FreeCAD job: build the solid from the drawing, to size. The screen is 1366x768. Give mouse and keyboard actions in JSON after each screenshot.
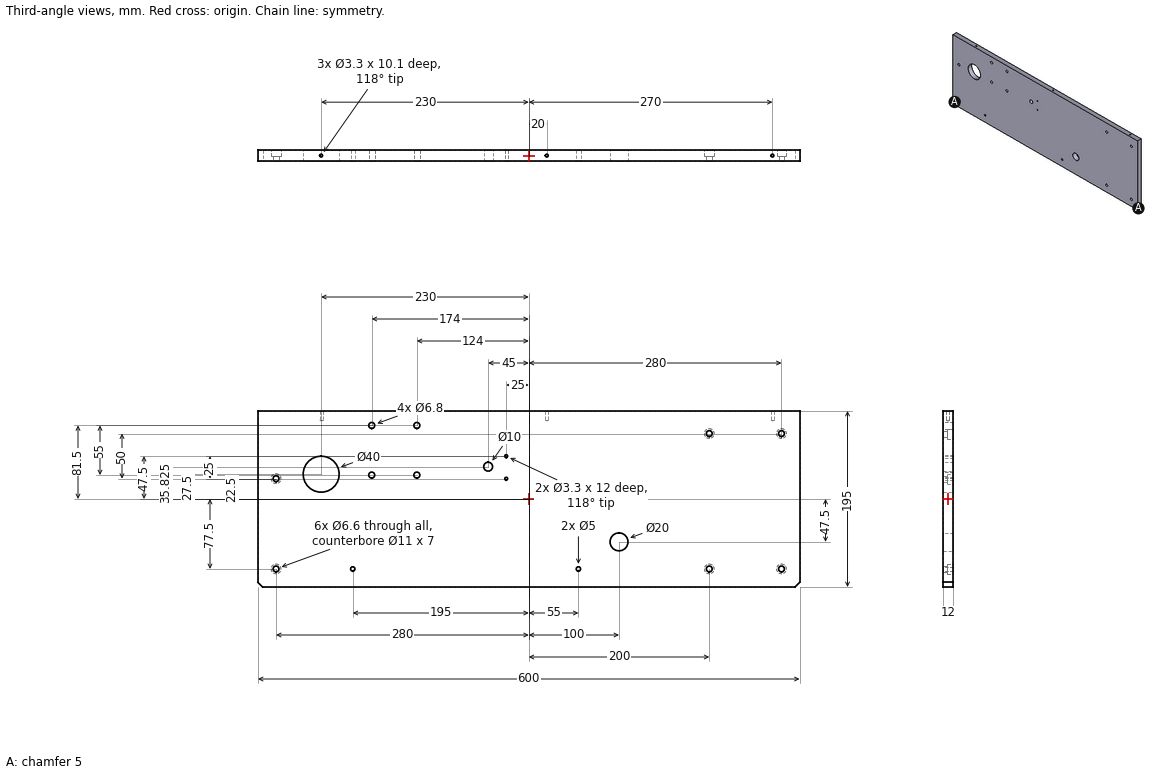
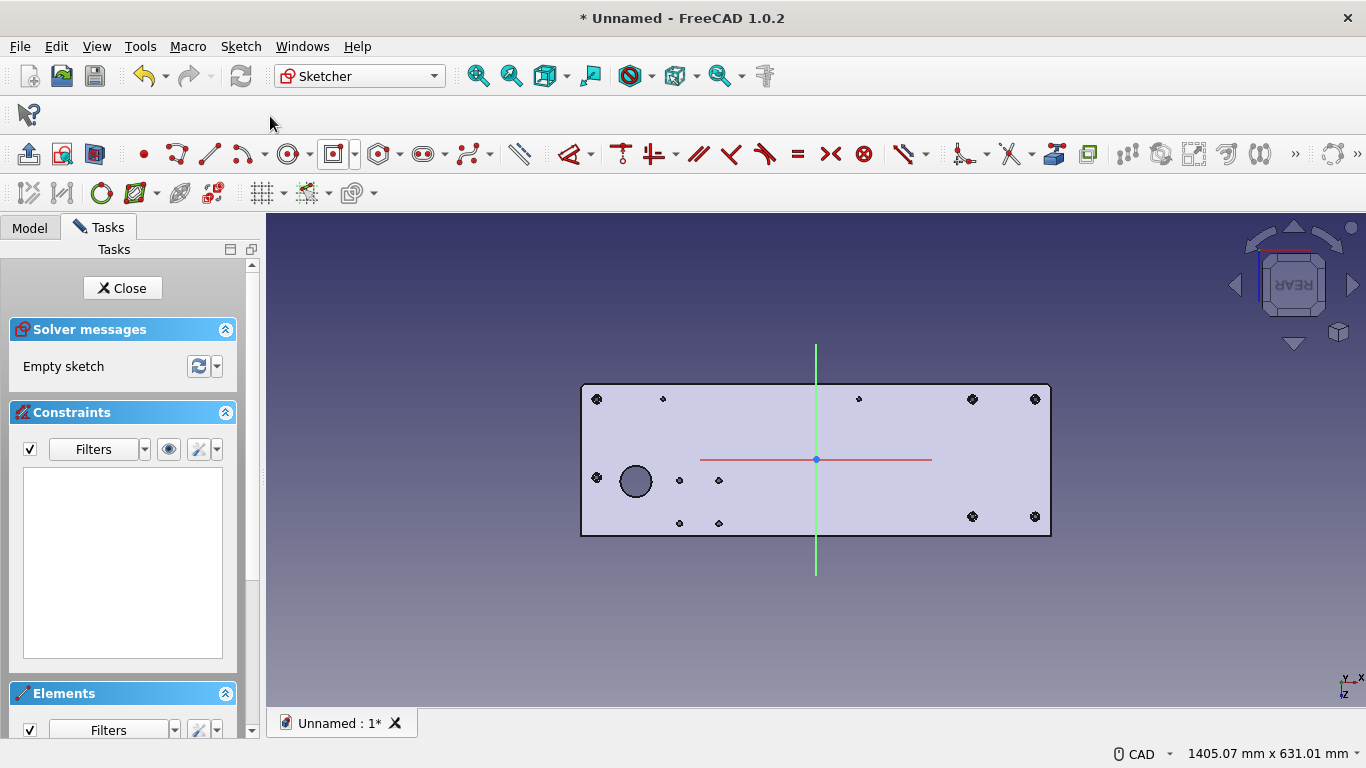
{"action": "scroll", "coordinate": [902, 421], "scroll_direction": "up", "scroll_amount": 15}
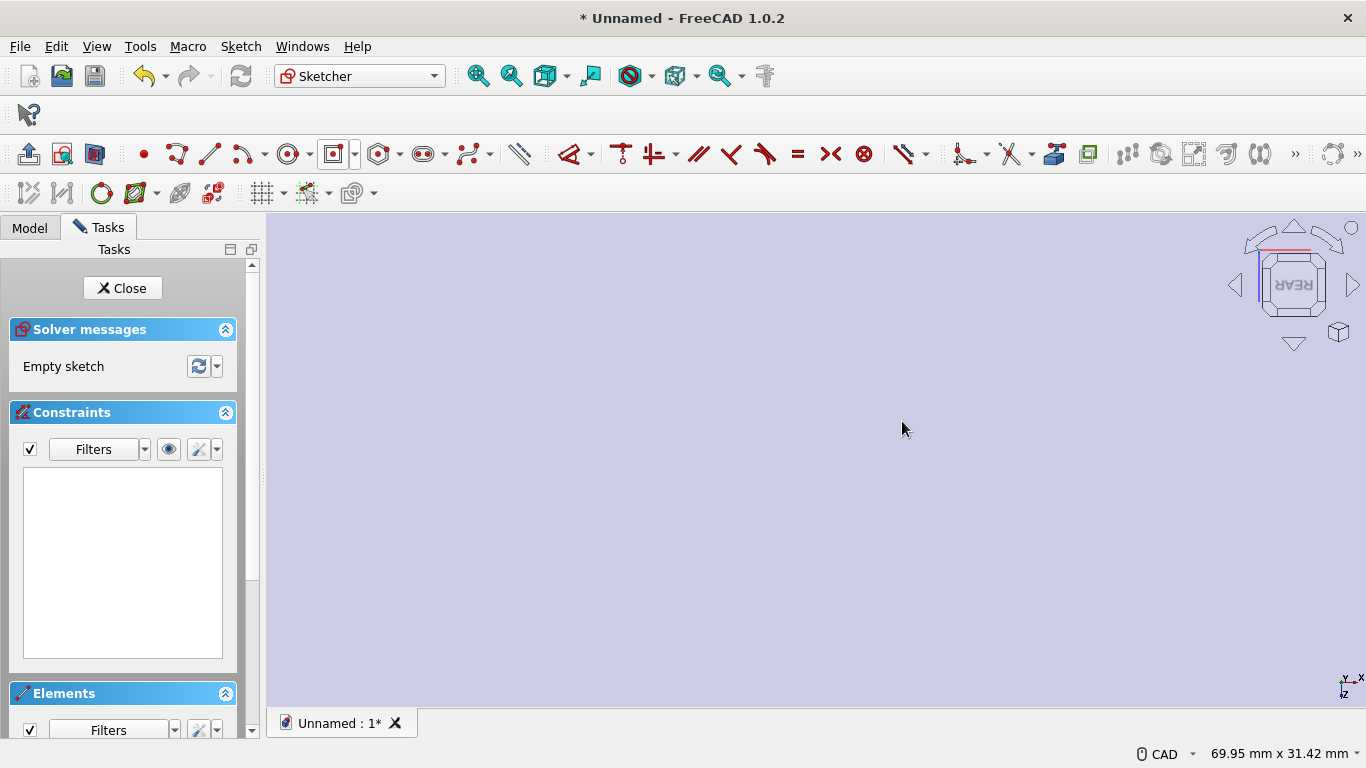
{"action": "key", "text": "g c"}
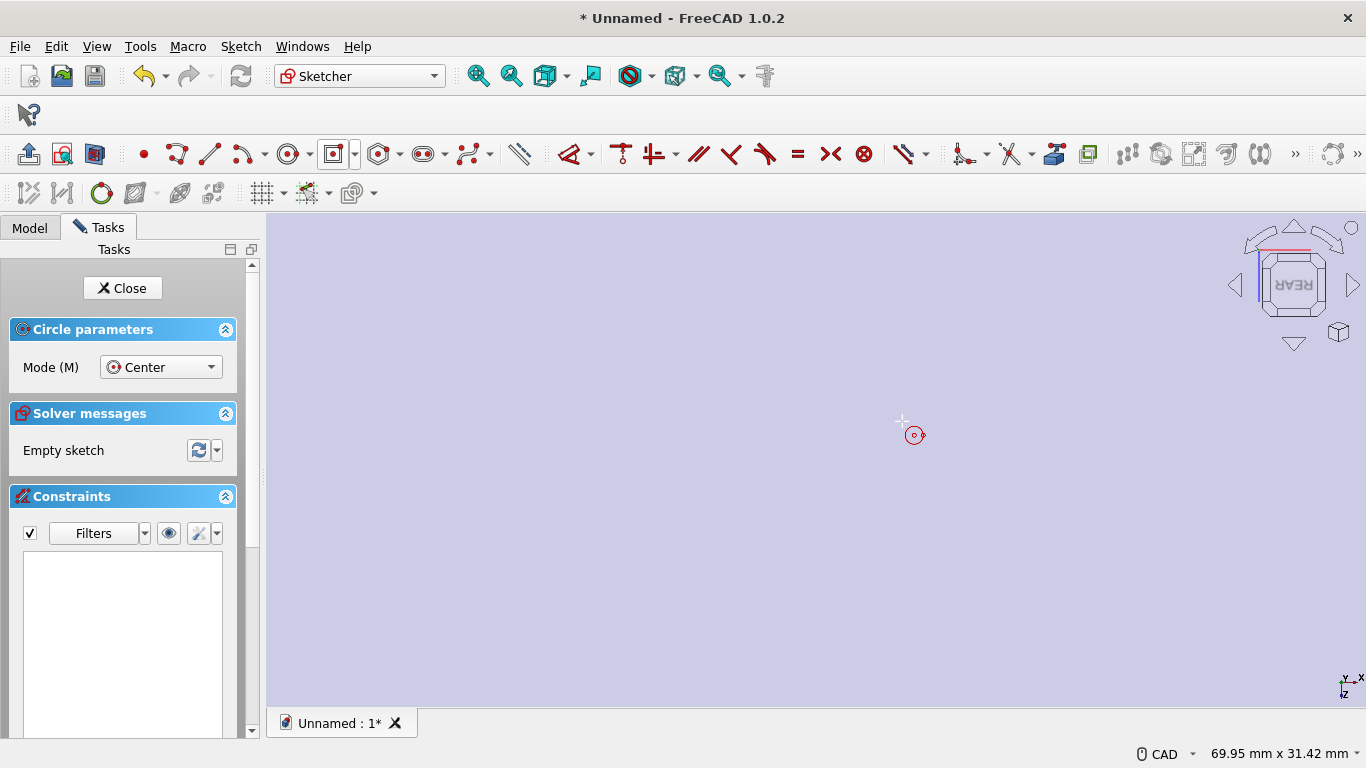
{"action": "left_click", "coordinate": [736, 449]}
{"action": "left_click", "coordinate": [847, 338]}
{"action": "key", "text": "Escape"}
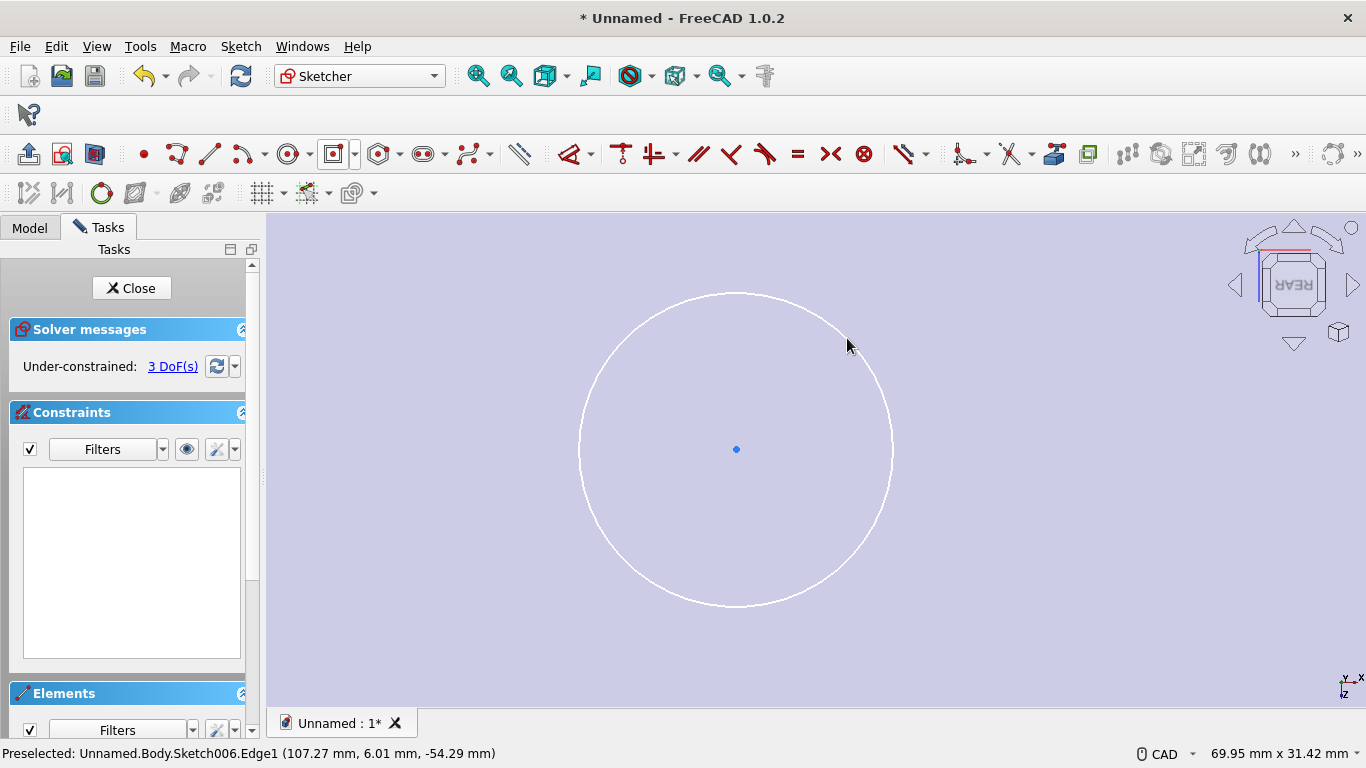
{"action": "key", "text": "d"}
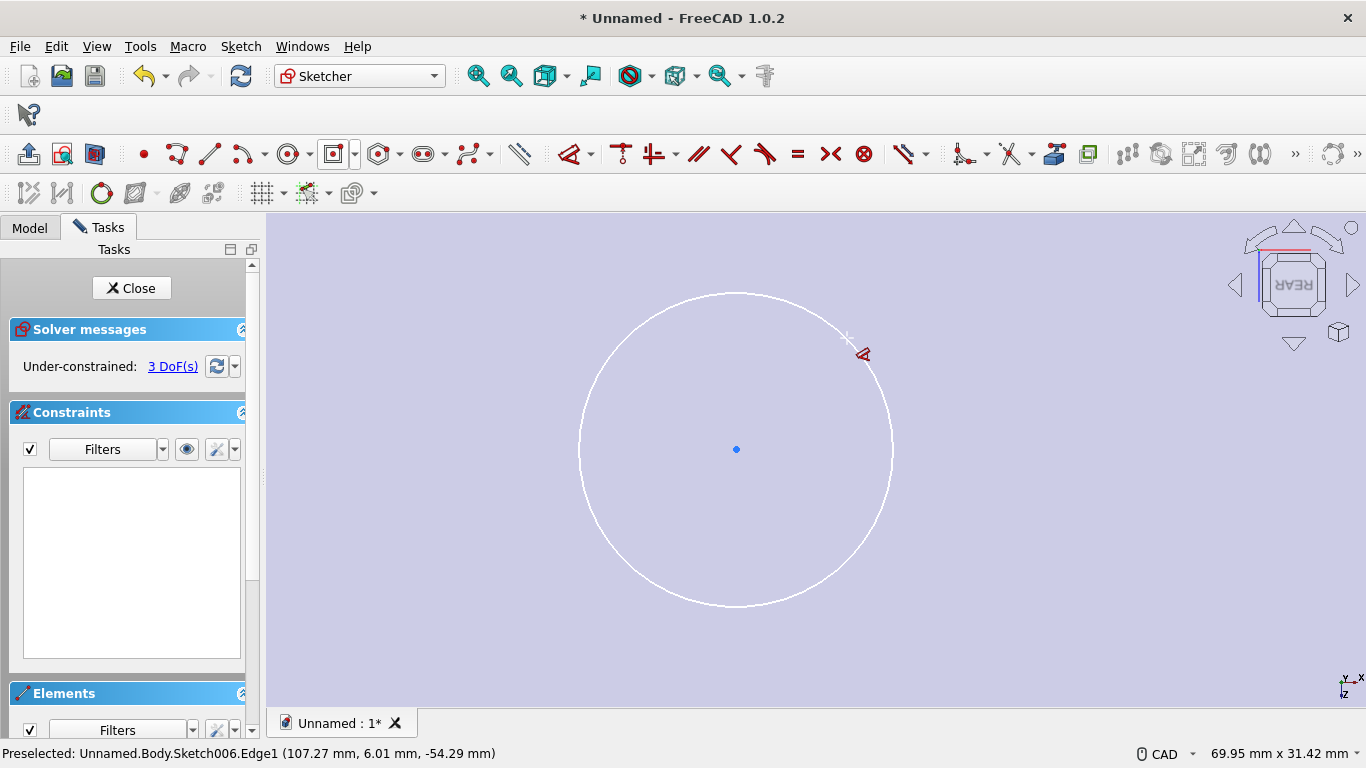
{"action": "left_click", "coordinate": [847, 339]}
{"action": "left_click", "coordinate": [870, 316]}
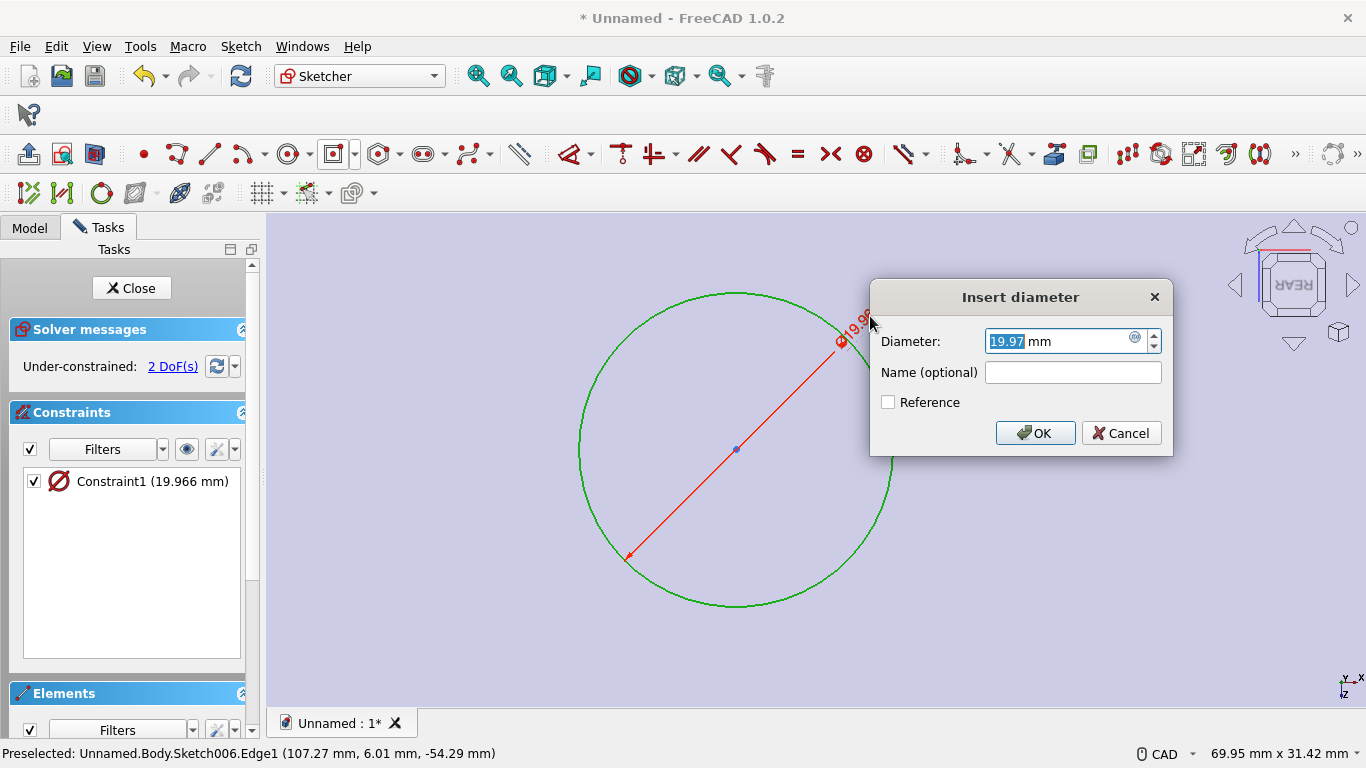
{"action": "type", "text": "20"}
{"action": "key", "text": "Return"}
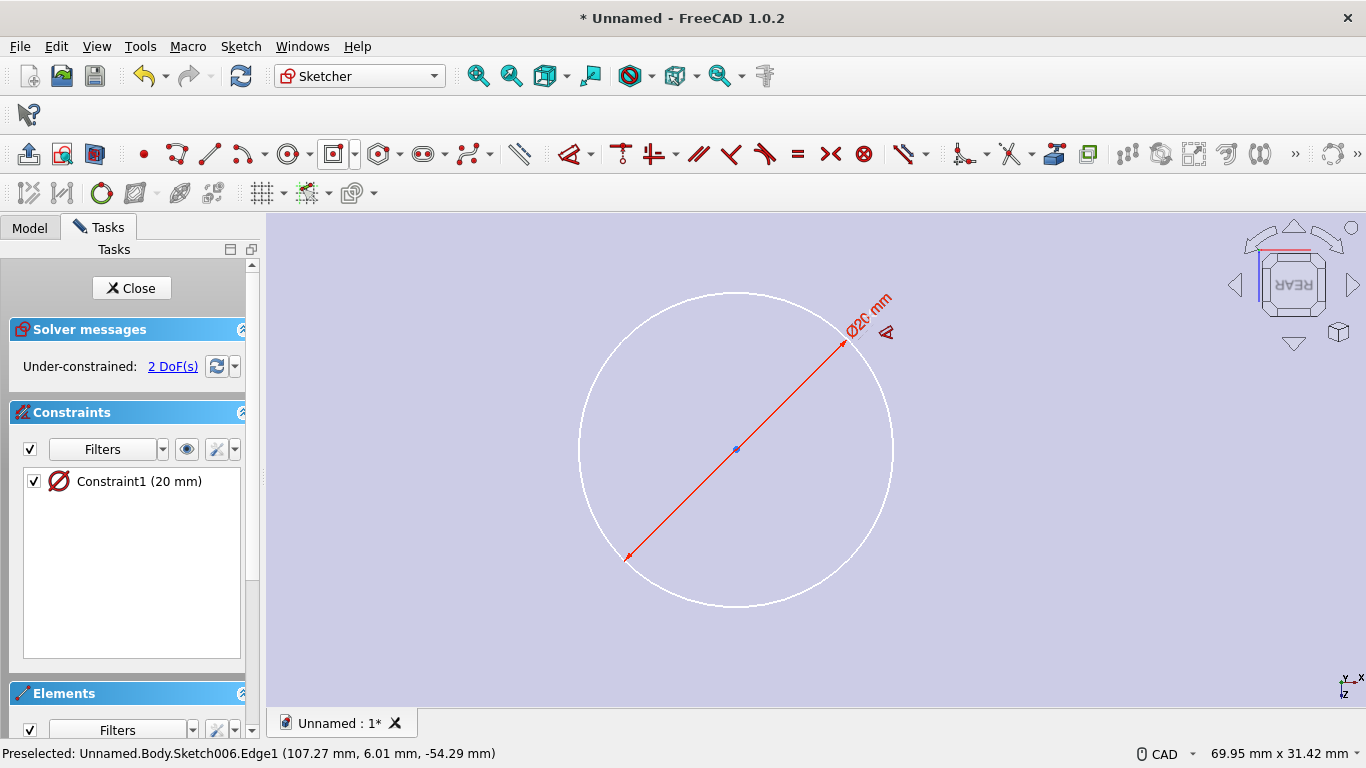
{"action": "left_click", "coordinate": [736, 450]}
{"action": "left_click", "coordinate": [515, 416]}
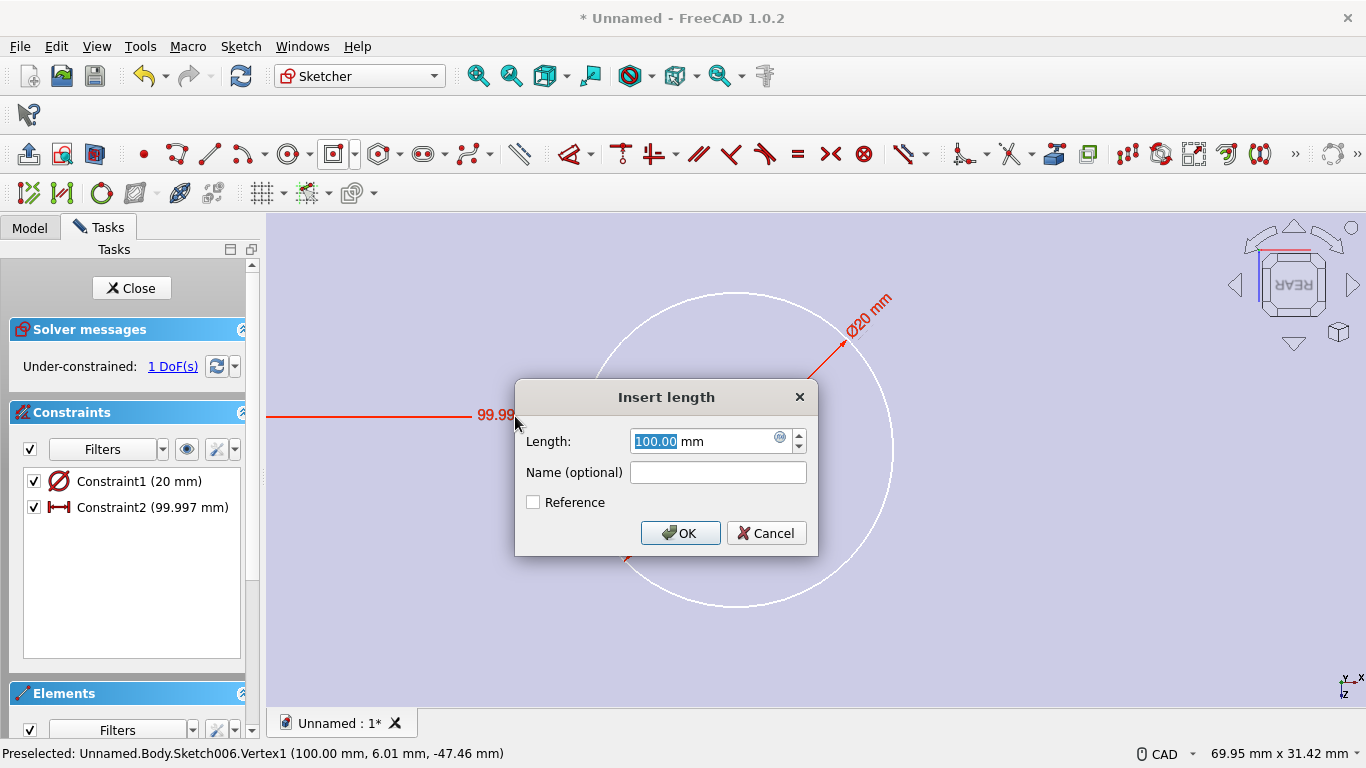
{"action": "type", "text": "100"}
{"action": "key", "text": "Return"}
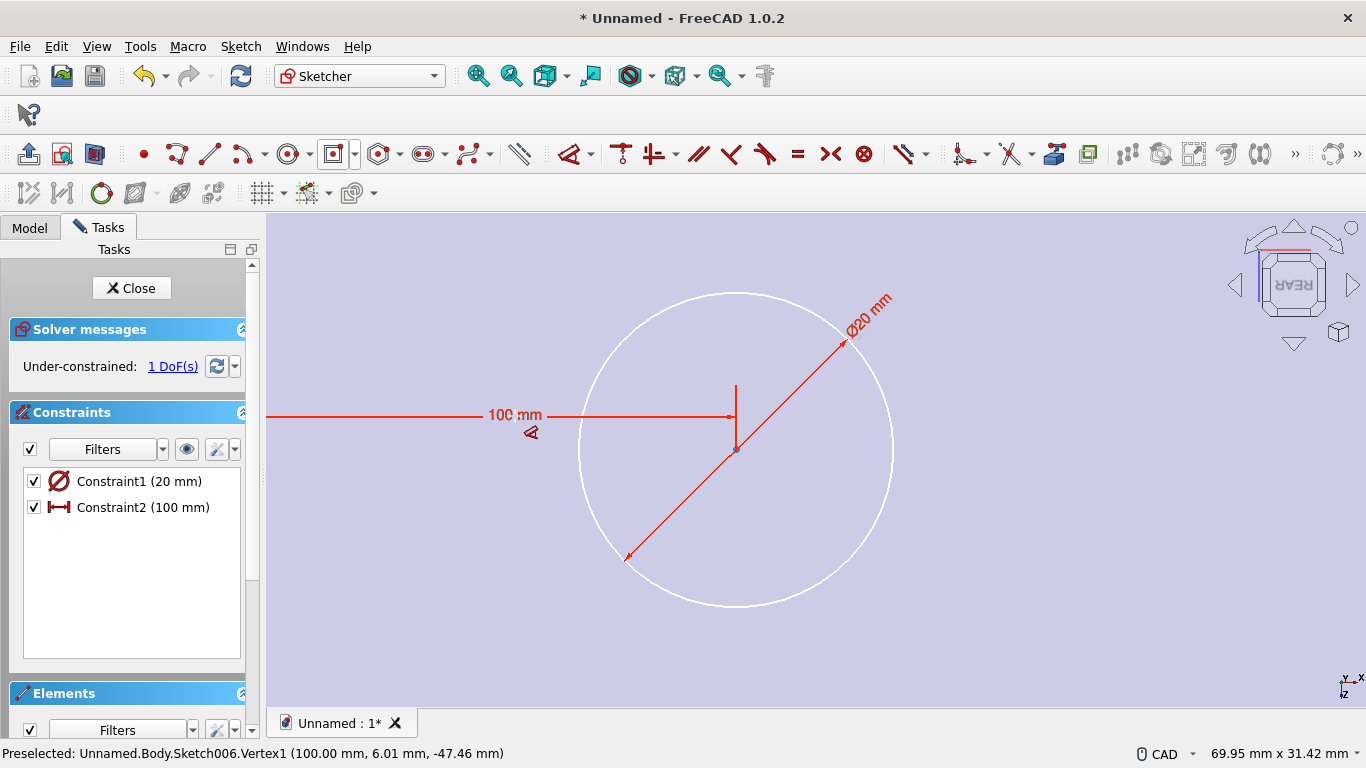
{"action": "left_click", "coordinate": [736, 450]}
{"action": "left_click", "coordinate": [770, 564]}